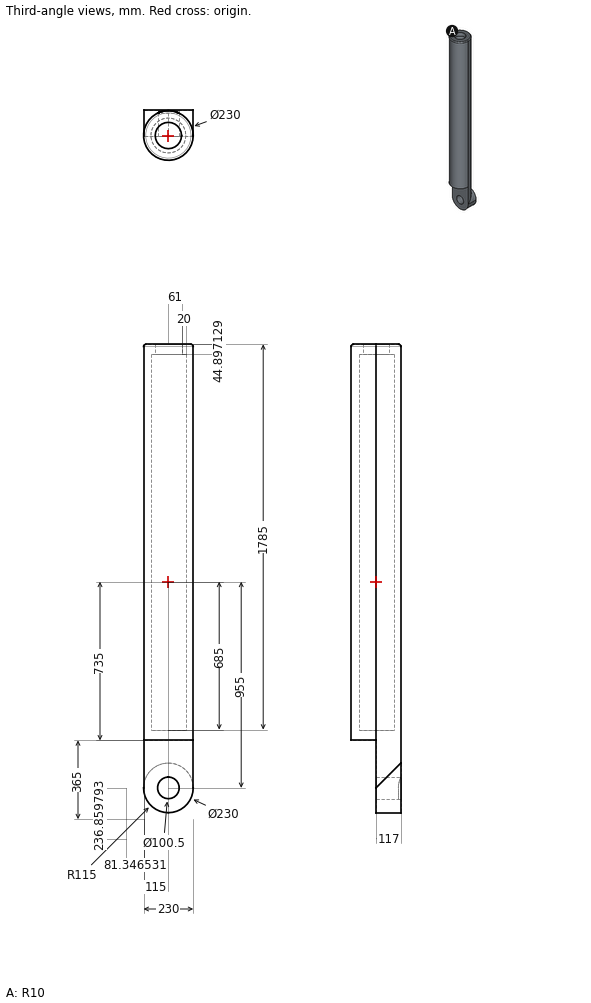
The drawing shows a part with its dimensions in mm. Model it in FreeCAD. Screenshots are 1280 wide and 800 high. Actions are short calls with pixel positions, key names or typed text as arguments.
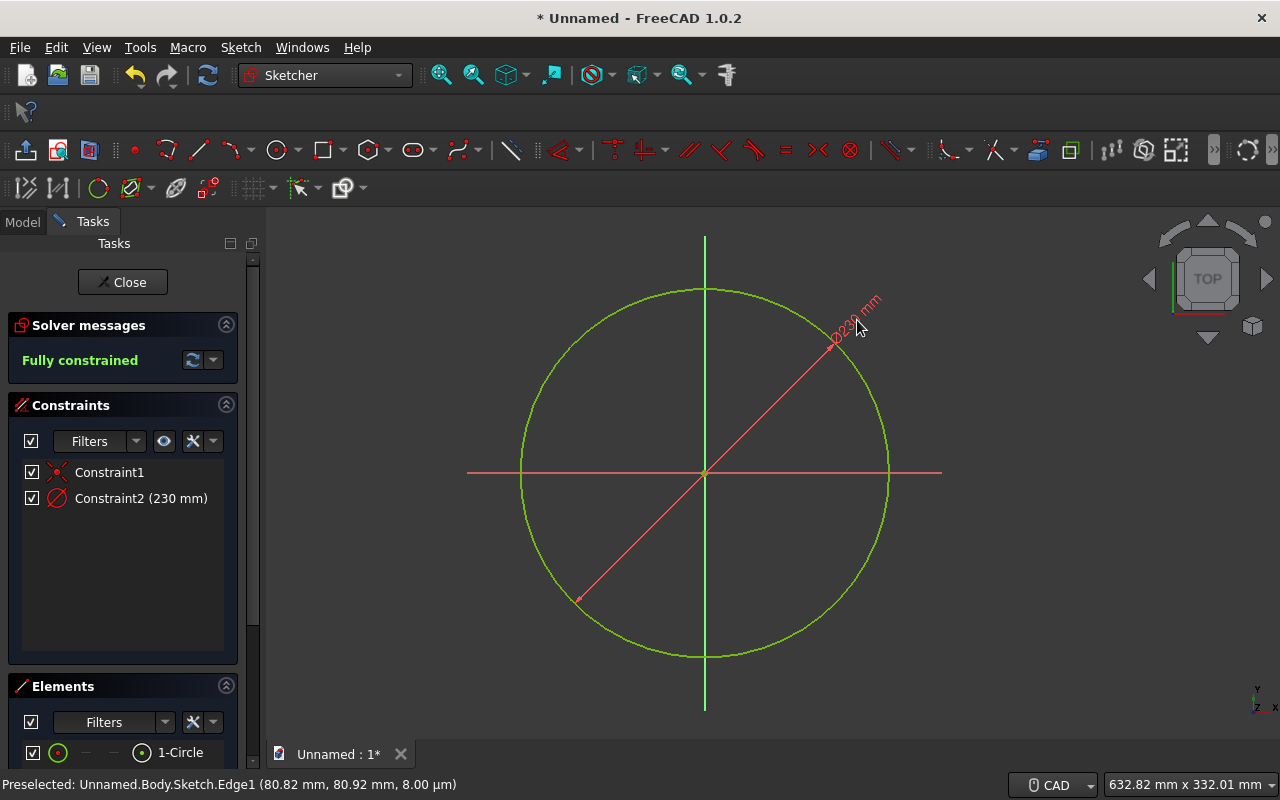
click(123, 282)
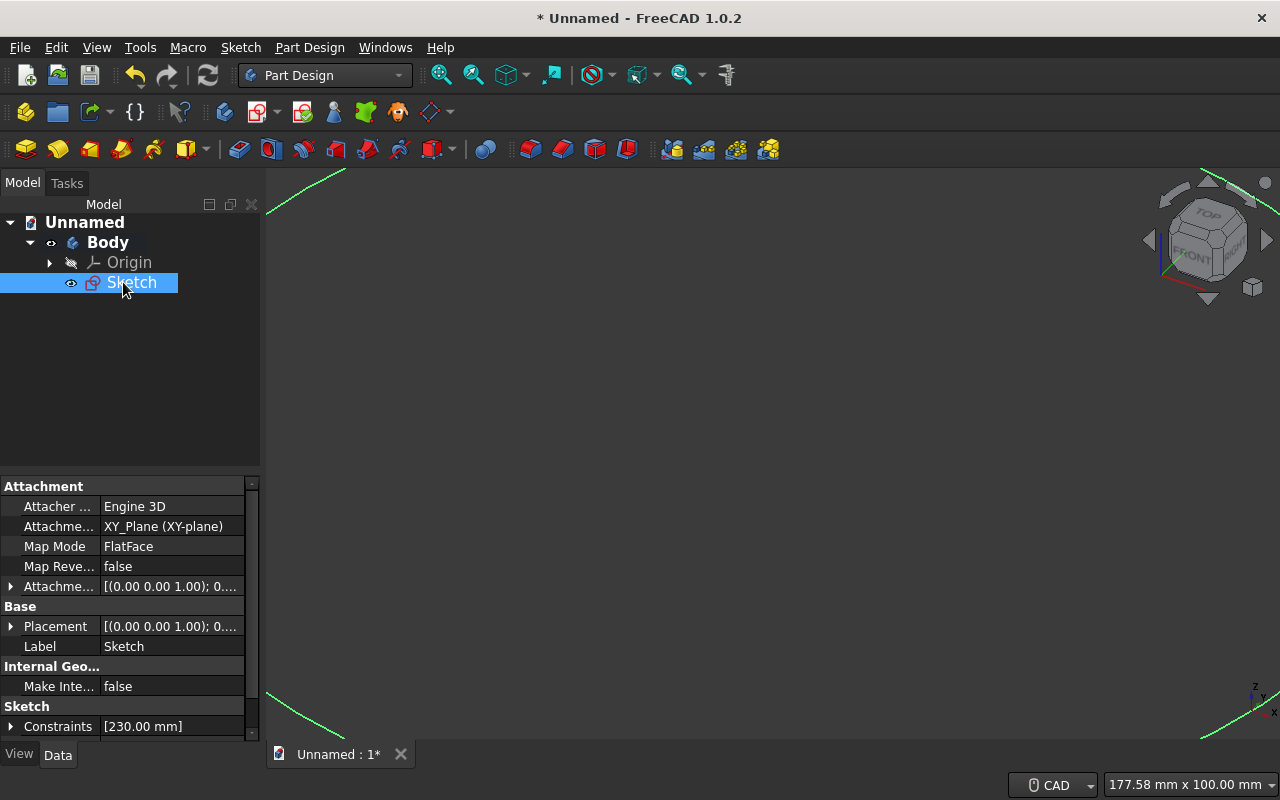
click(26, 150)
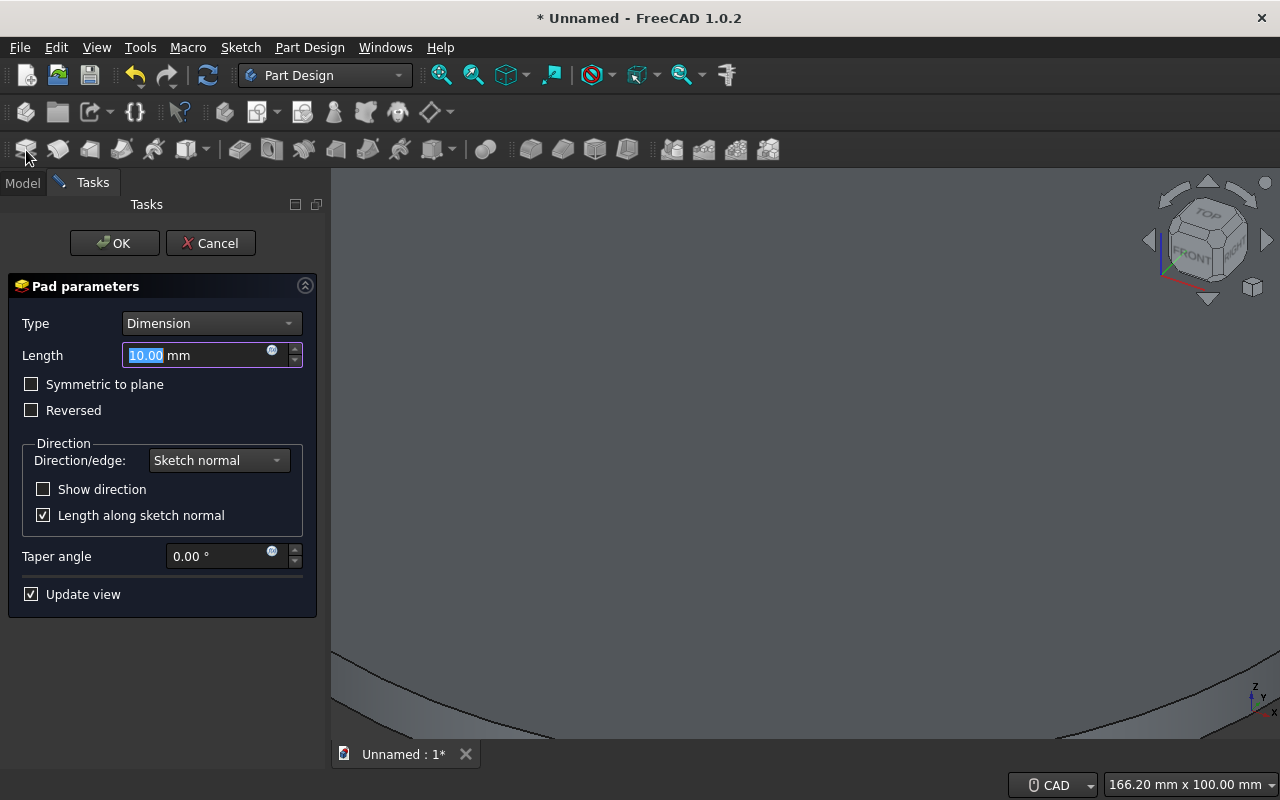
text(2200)
key(Tab)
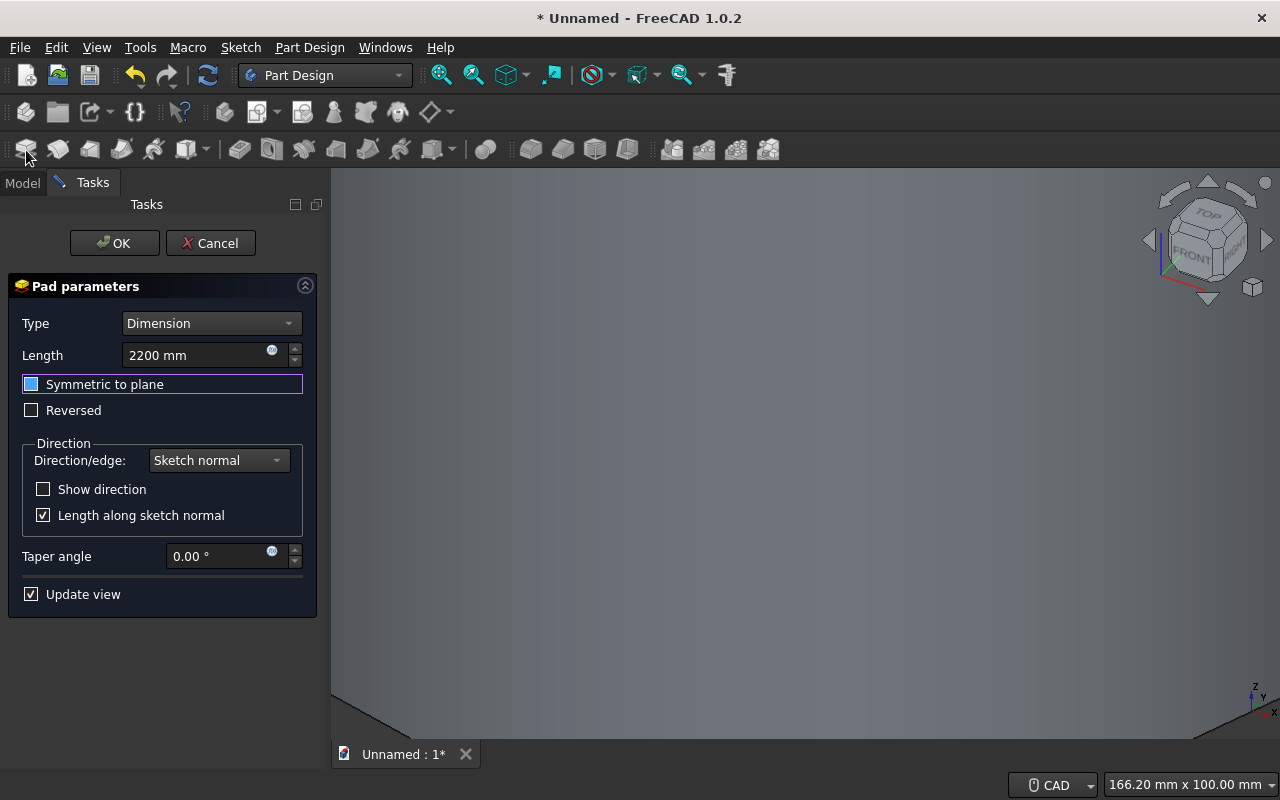
click(30, 384)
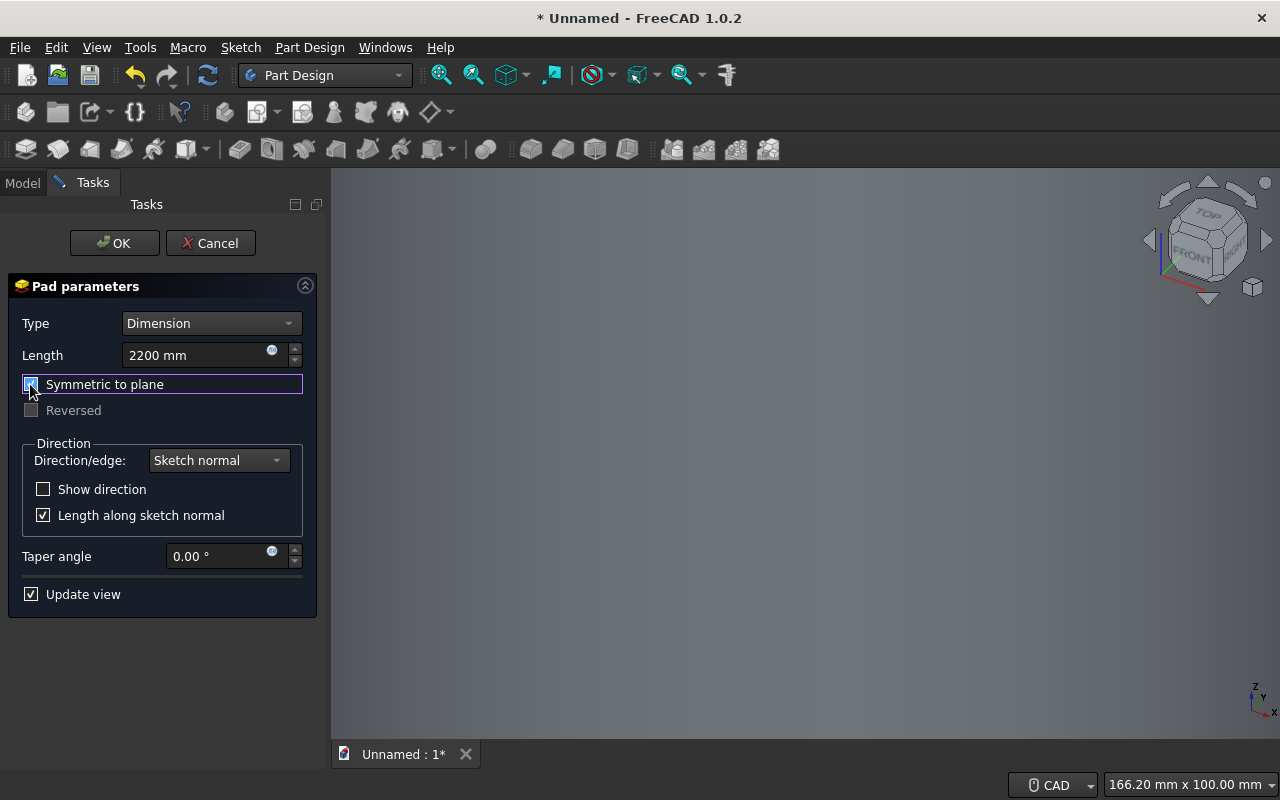
click(115, 243)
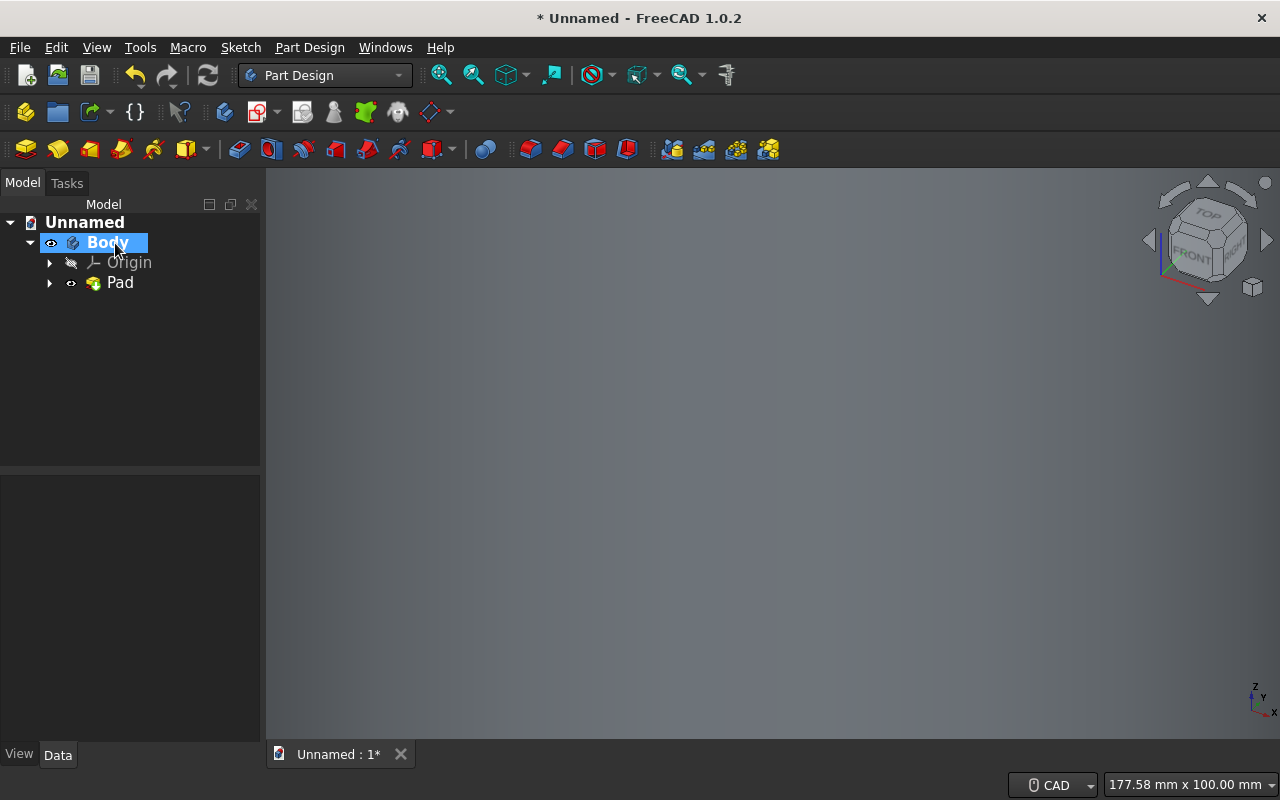
click(442, 76)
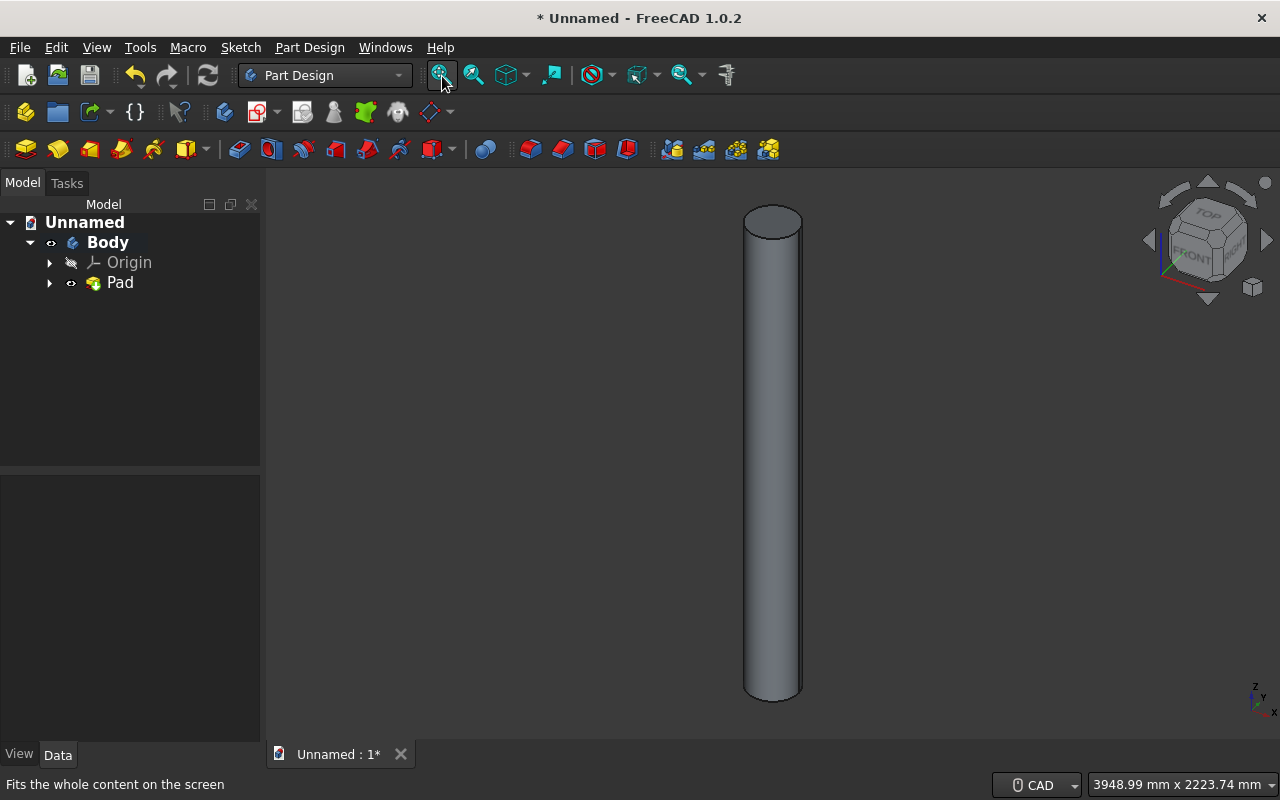
click(258, 112)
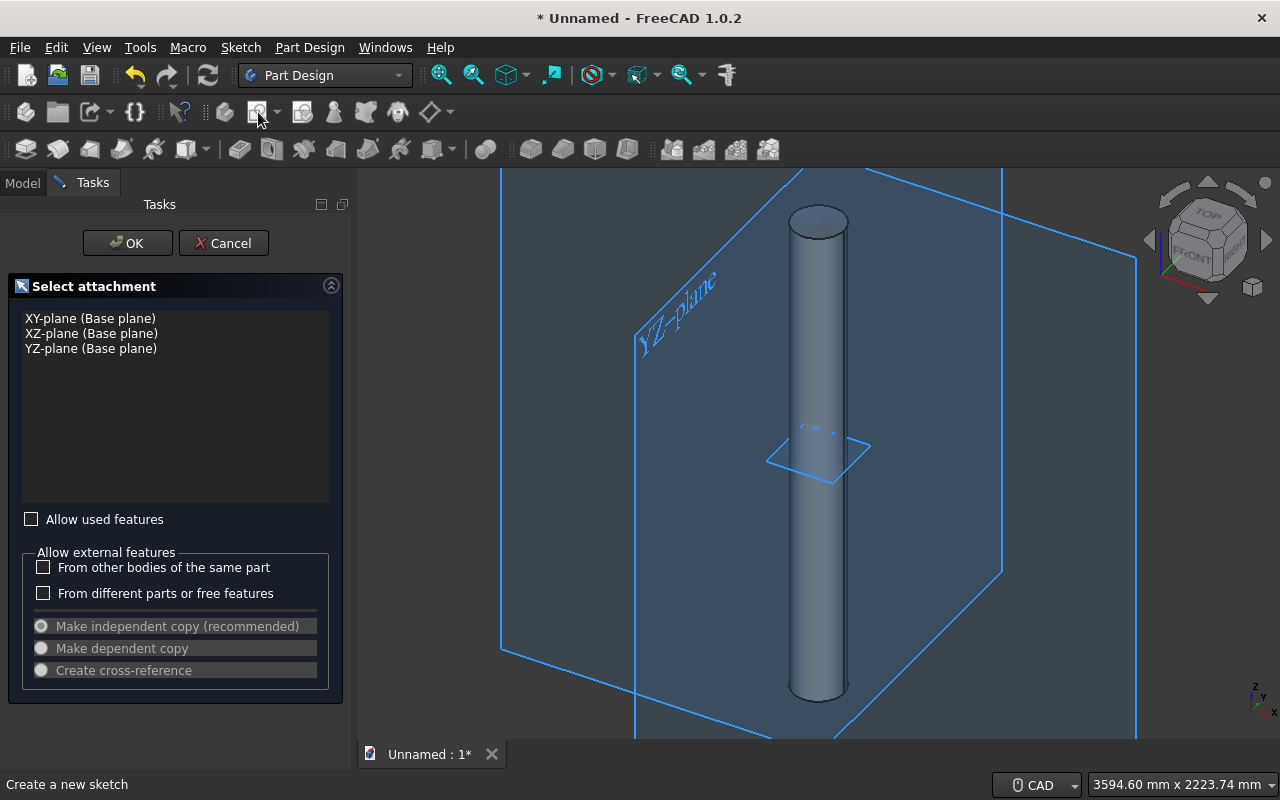
click(82, 334)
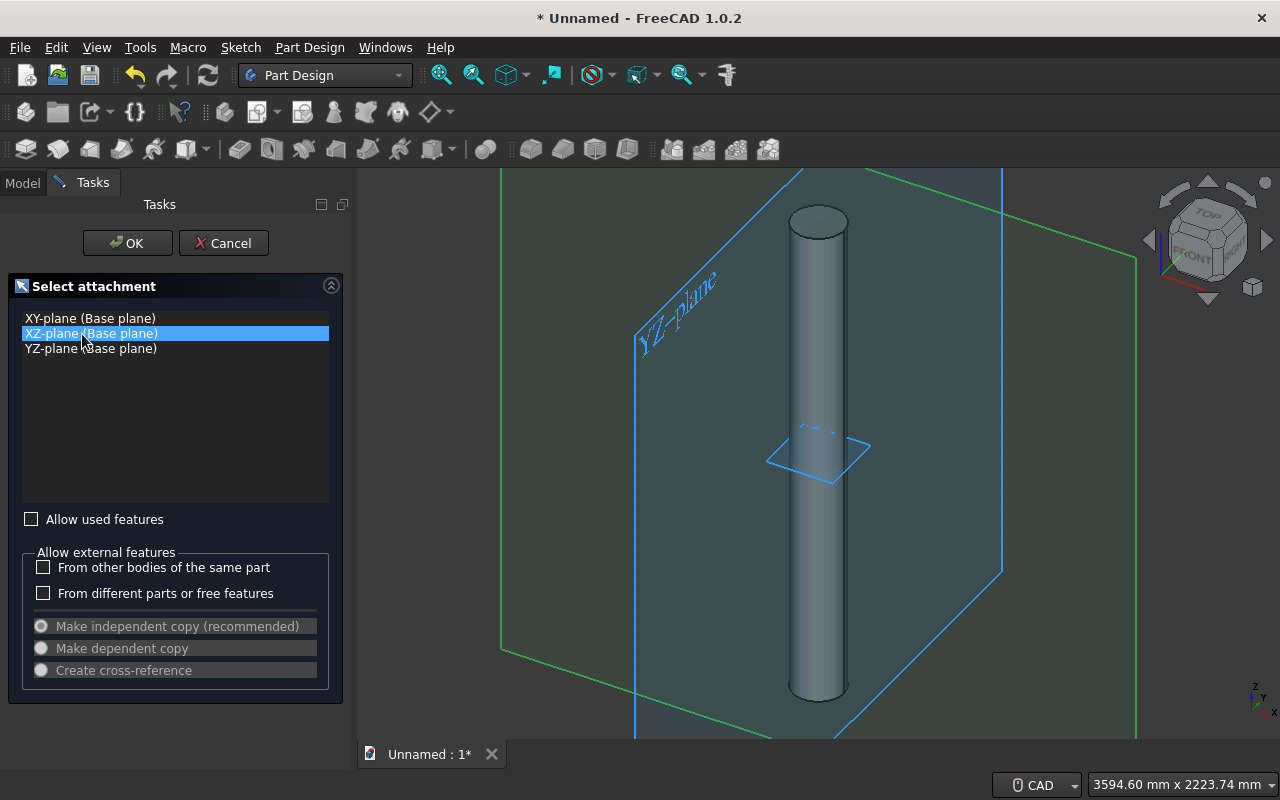
click(128, 243)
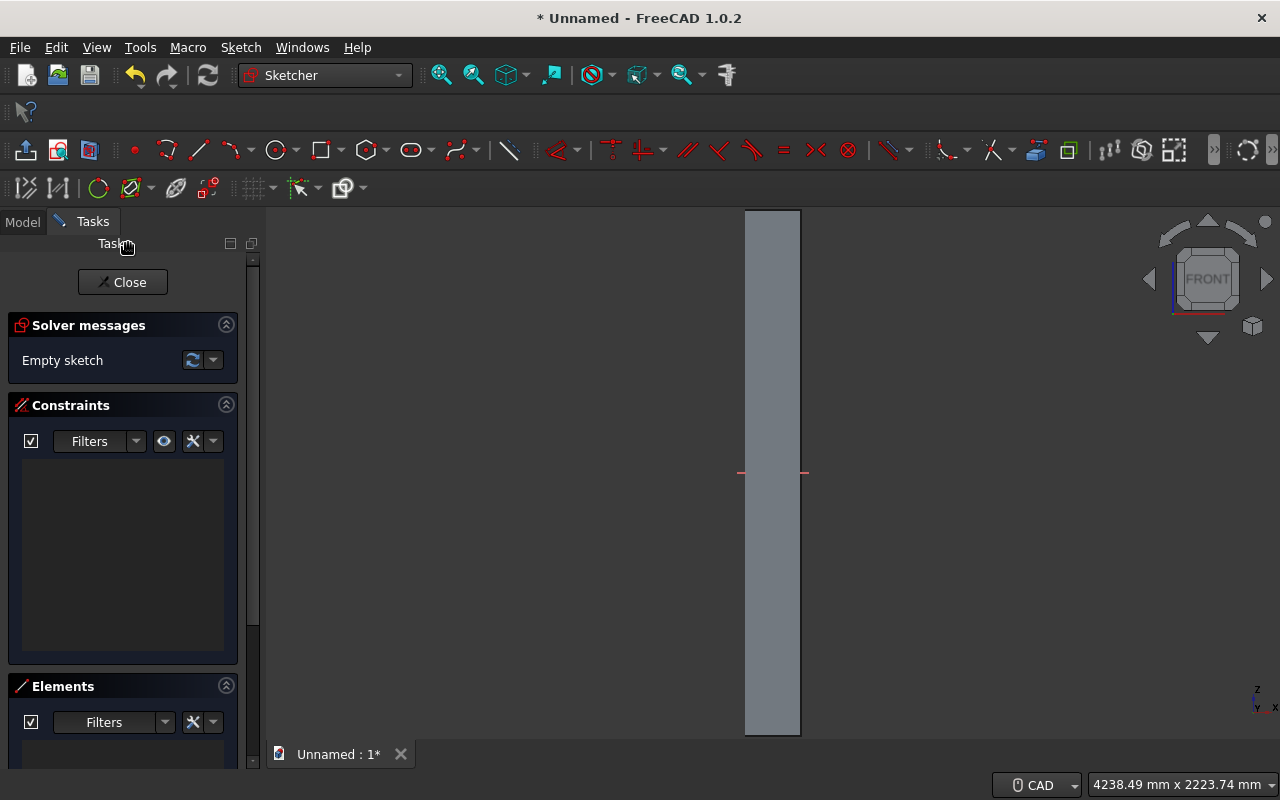
click(90, 150)